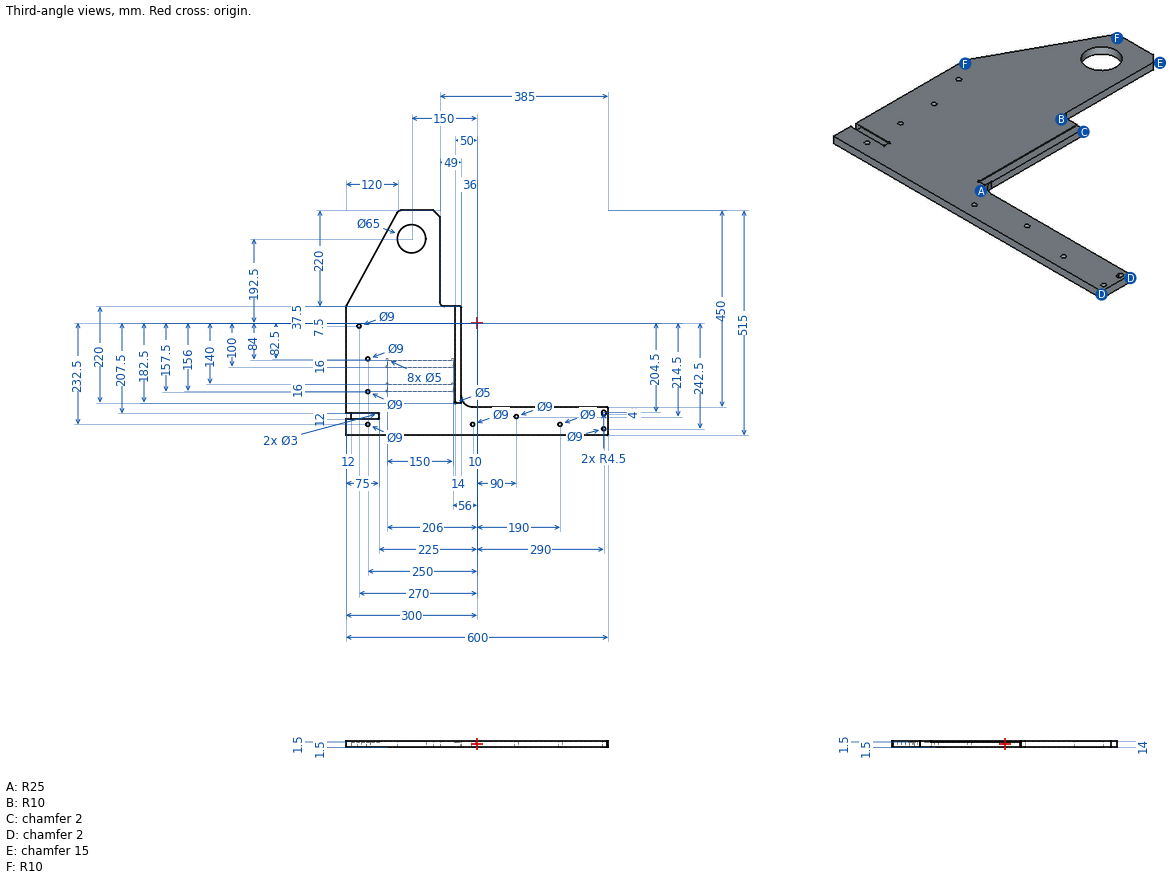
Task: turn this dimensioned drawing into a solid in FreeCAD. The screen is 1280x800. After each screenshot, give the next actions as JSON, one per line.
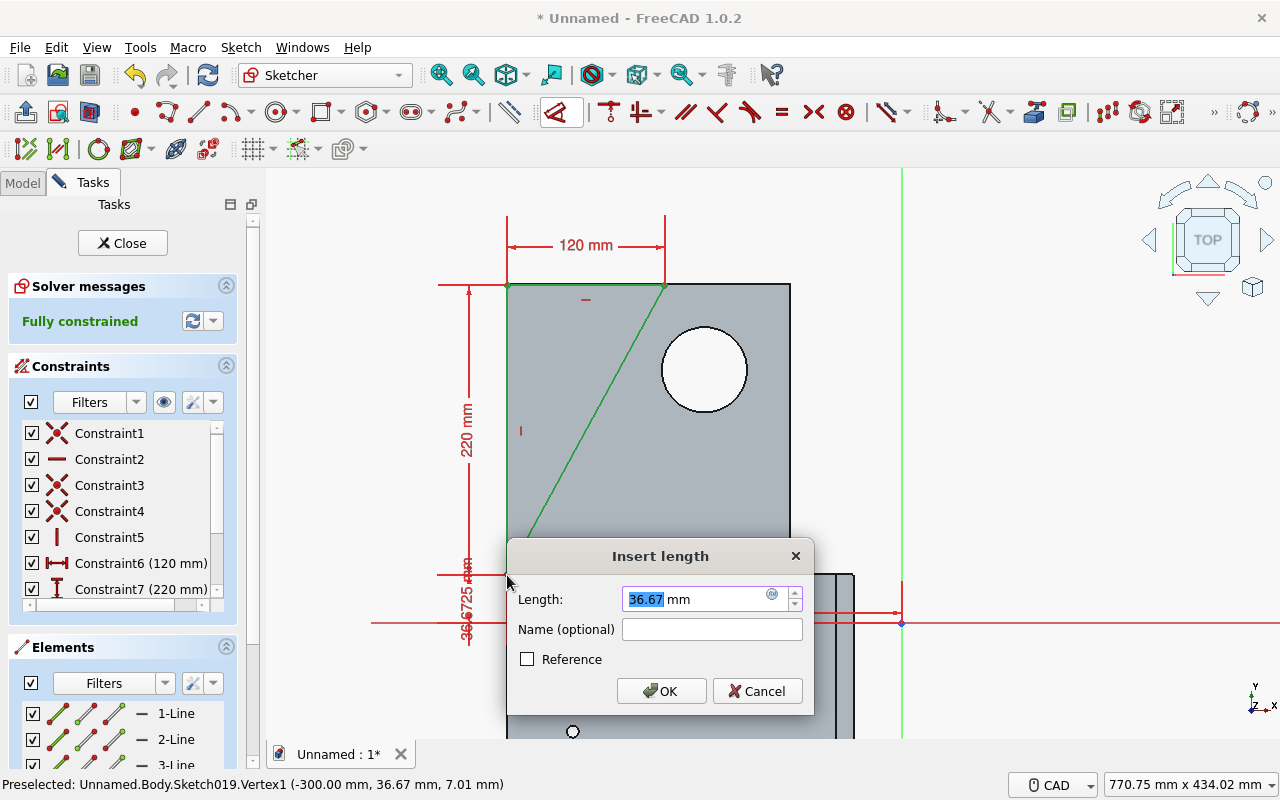
{"action": "type", "text": "37.5"}
{"action": "key", "text": "Return"}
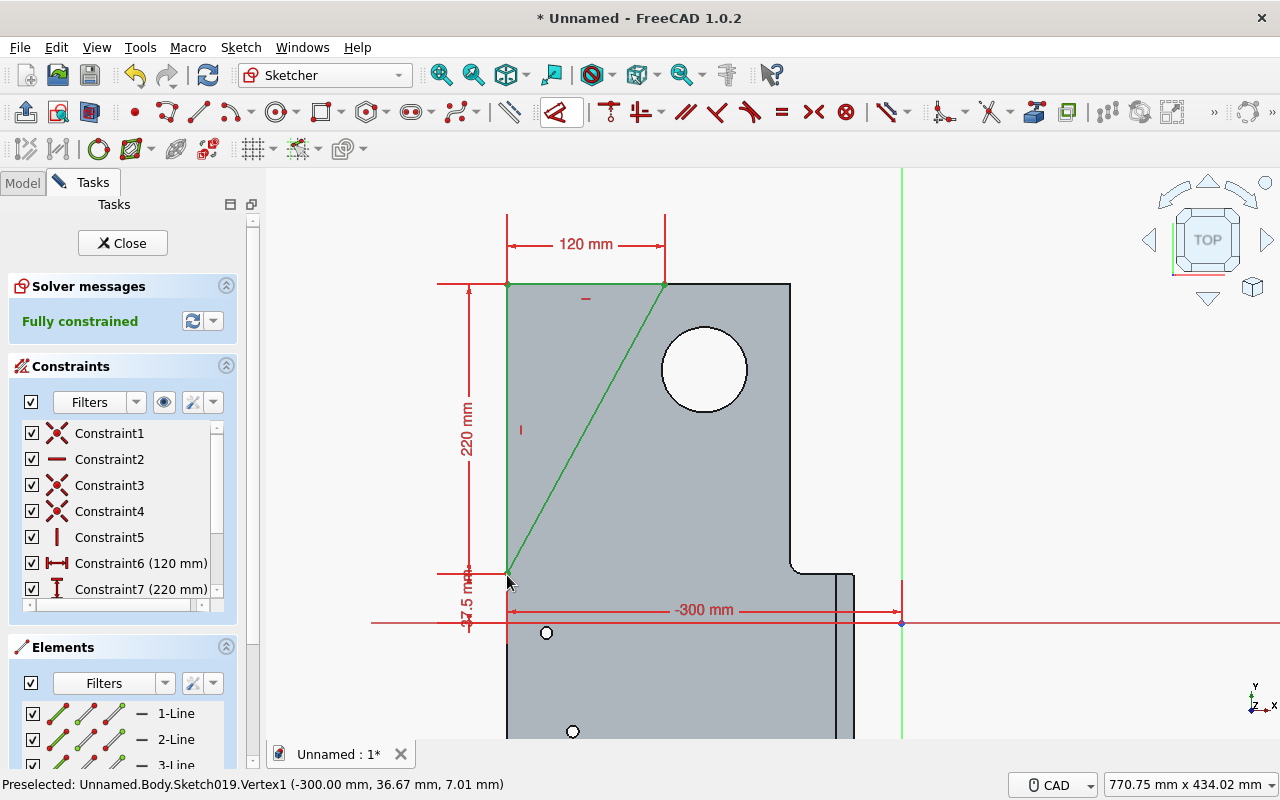
{"action": "left_click", "coordinate": [123, 243]}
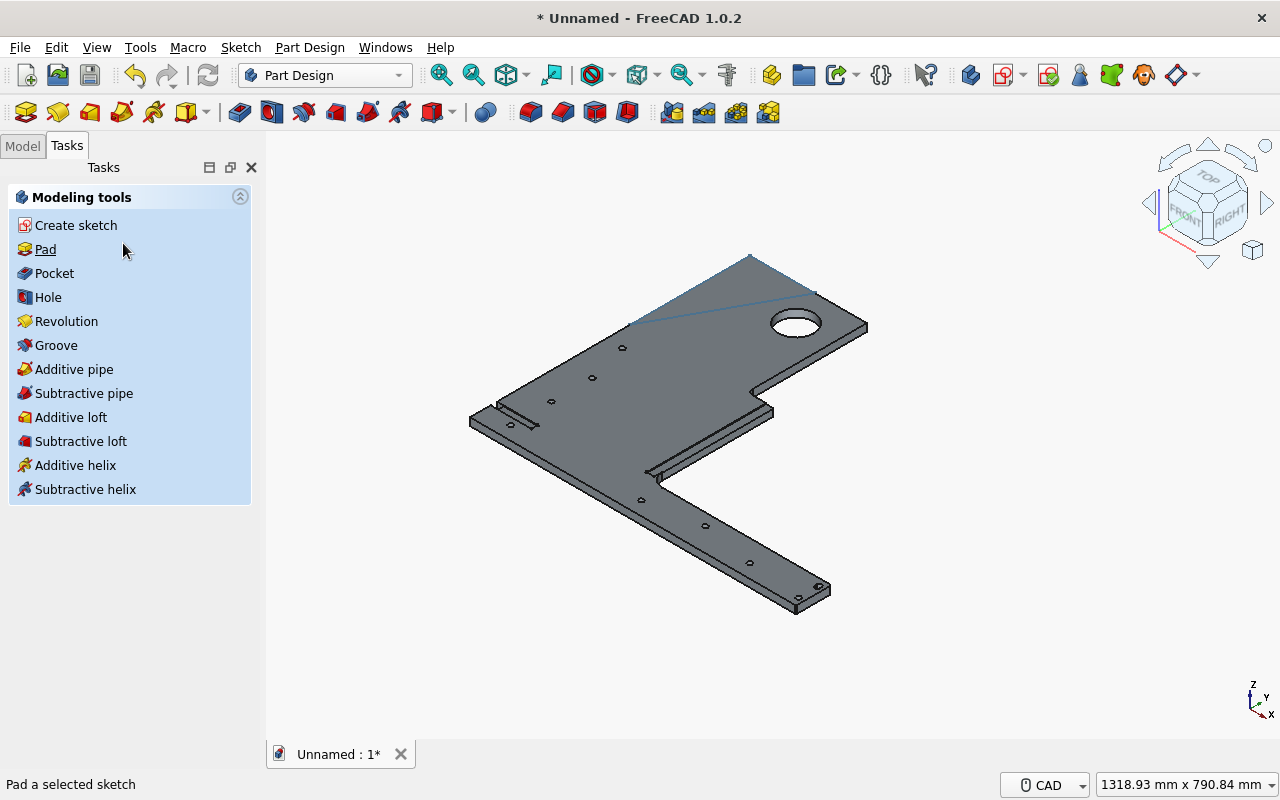
{"action": "left_click", "coordinate": [240, 112]}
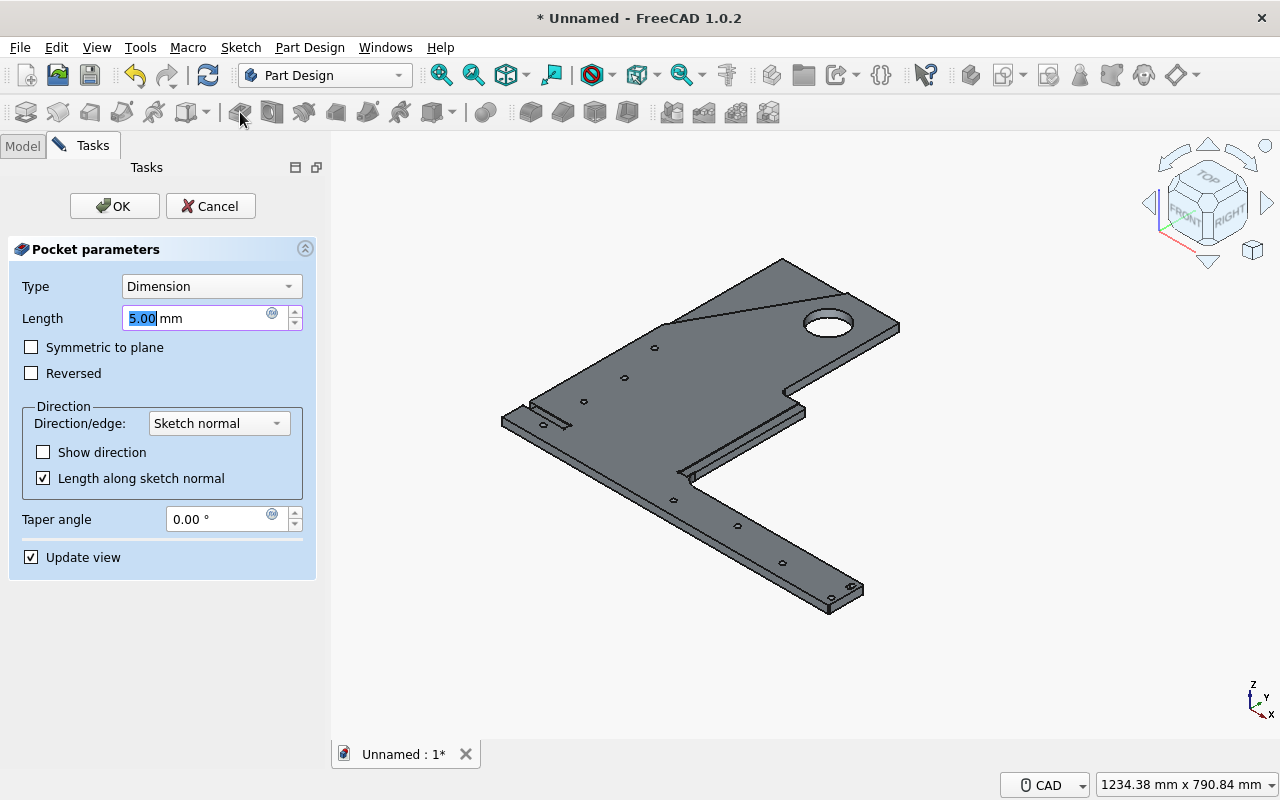
{"action": "left_click", "coordinate": [212, 286]}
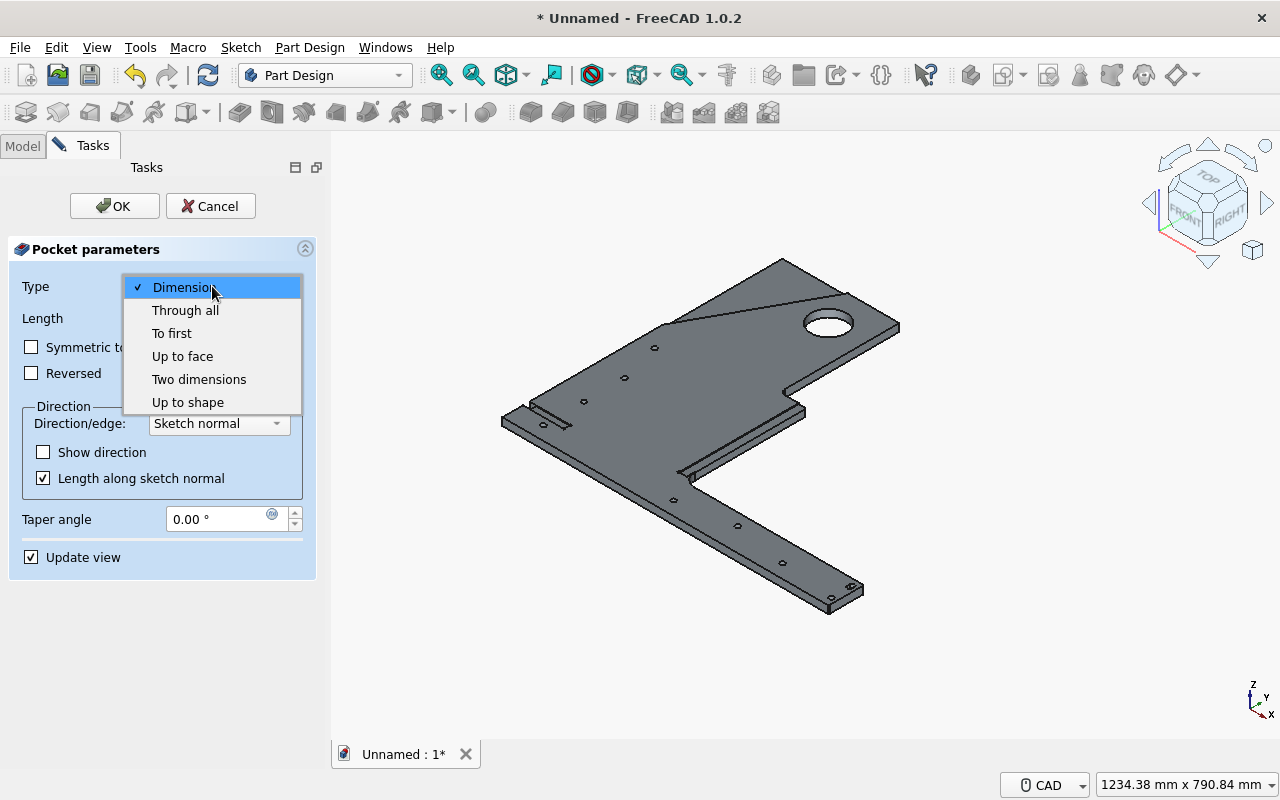
{"action": "left_click", "coordinate": [212, 334]}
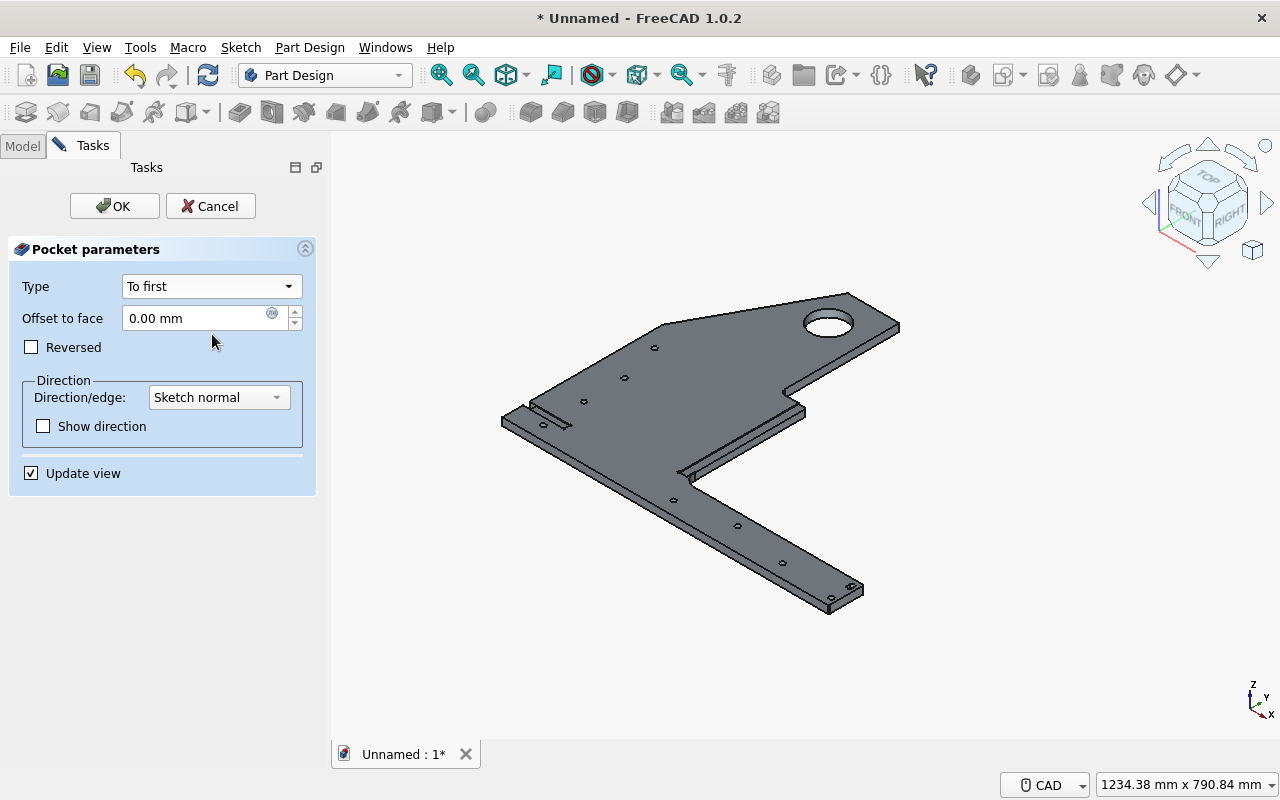
{"action": "left_click", "coordinate": [115, 206]}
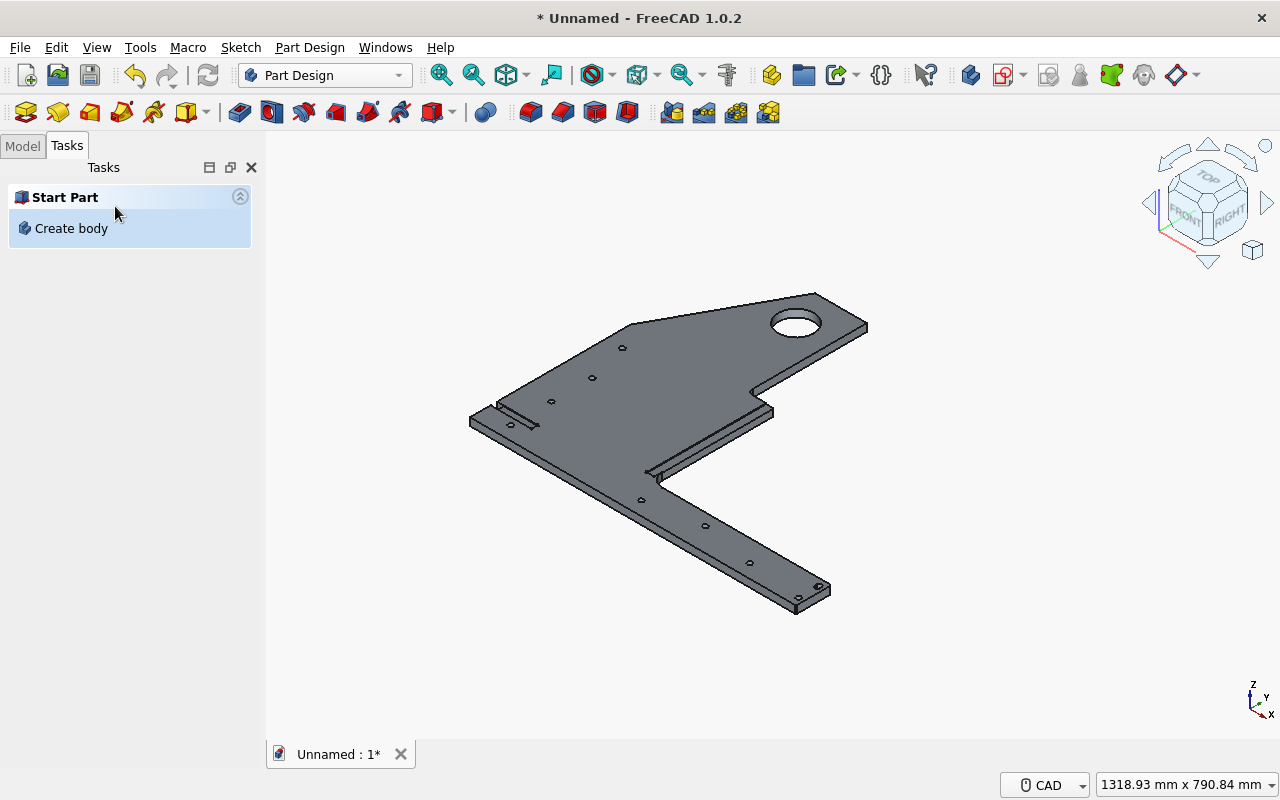
{"action": "scroll", "coordinate": [867, 327], "scroll_direction": "up", "scroll_amount": 7}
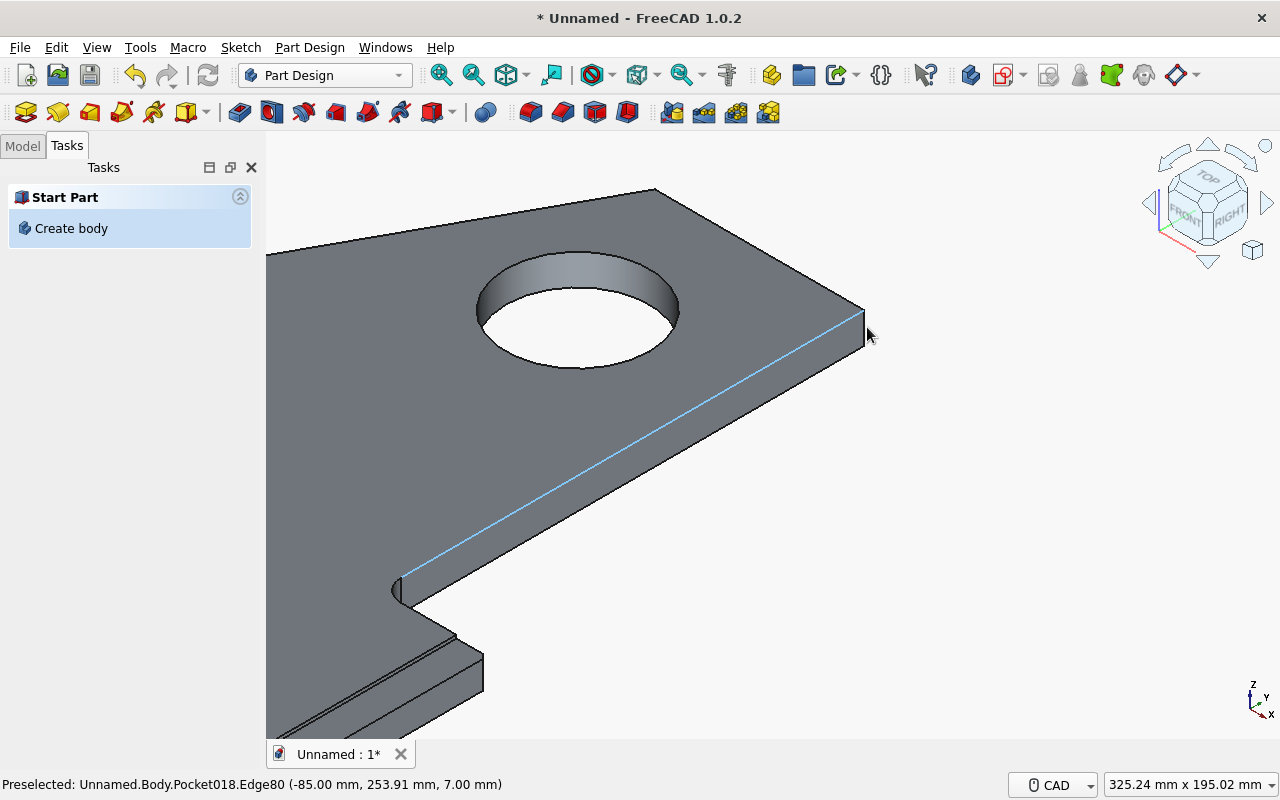
{"action": "left_click", "coordinate": [442, 76]}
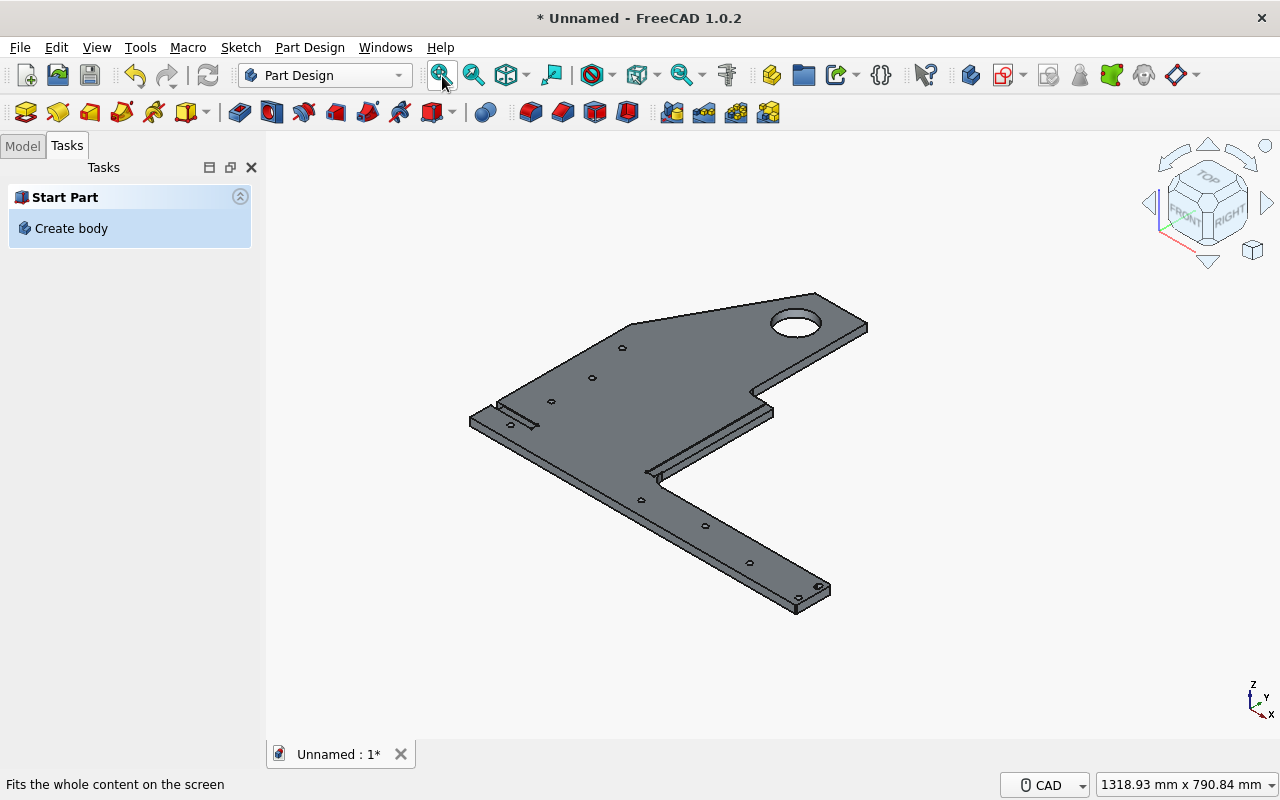
{"action": "key", "text": "2"}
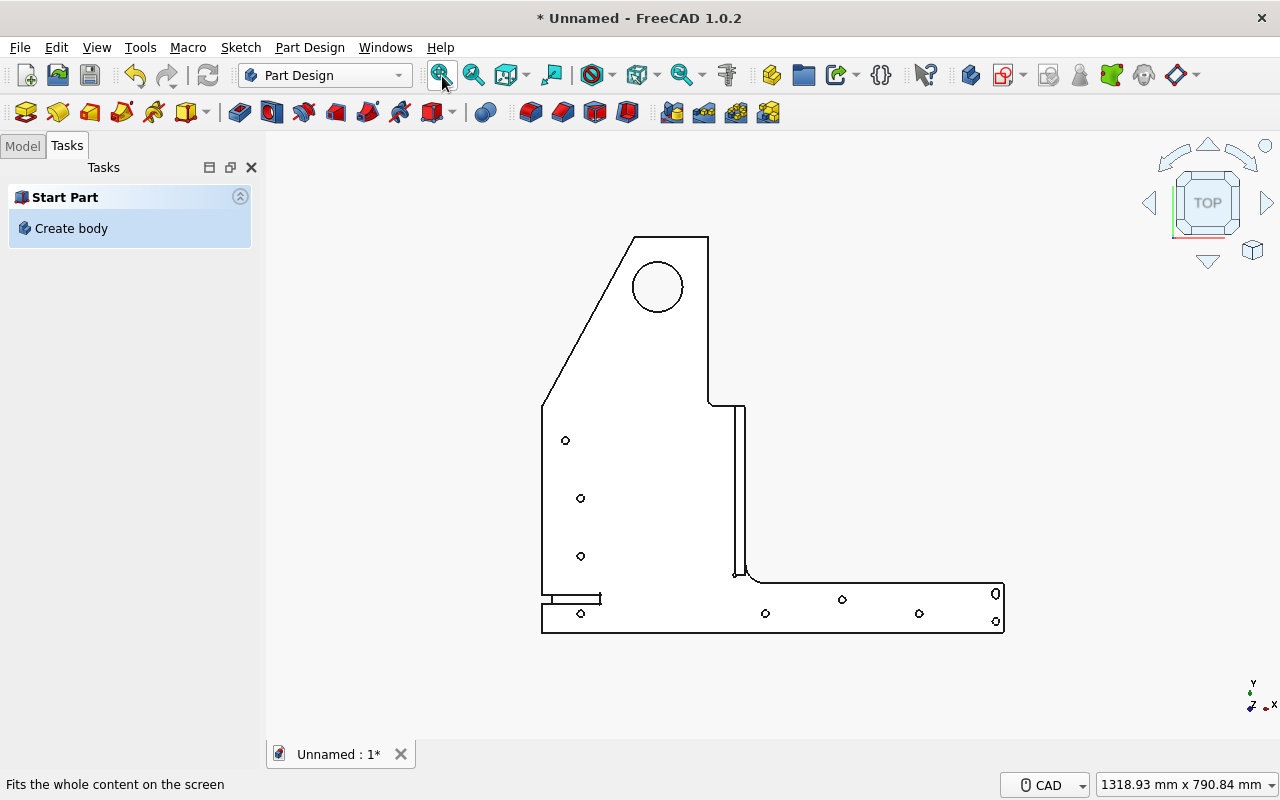
{"action": "scroll", "coordinate": [708, 236], "scroll_direction": "up", "scroll_amount": 7}